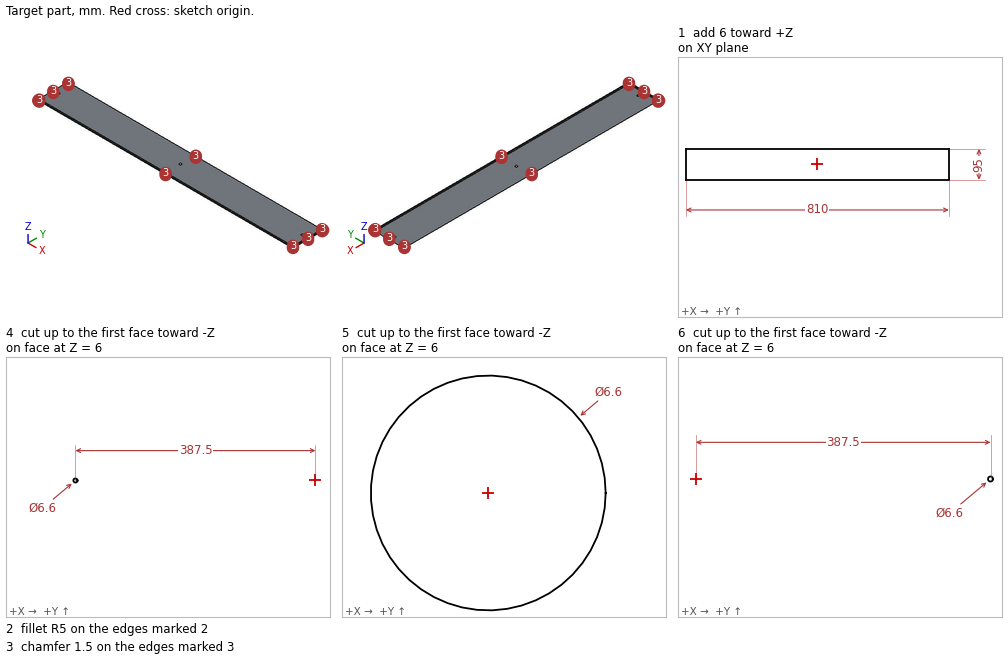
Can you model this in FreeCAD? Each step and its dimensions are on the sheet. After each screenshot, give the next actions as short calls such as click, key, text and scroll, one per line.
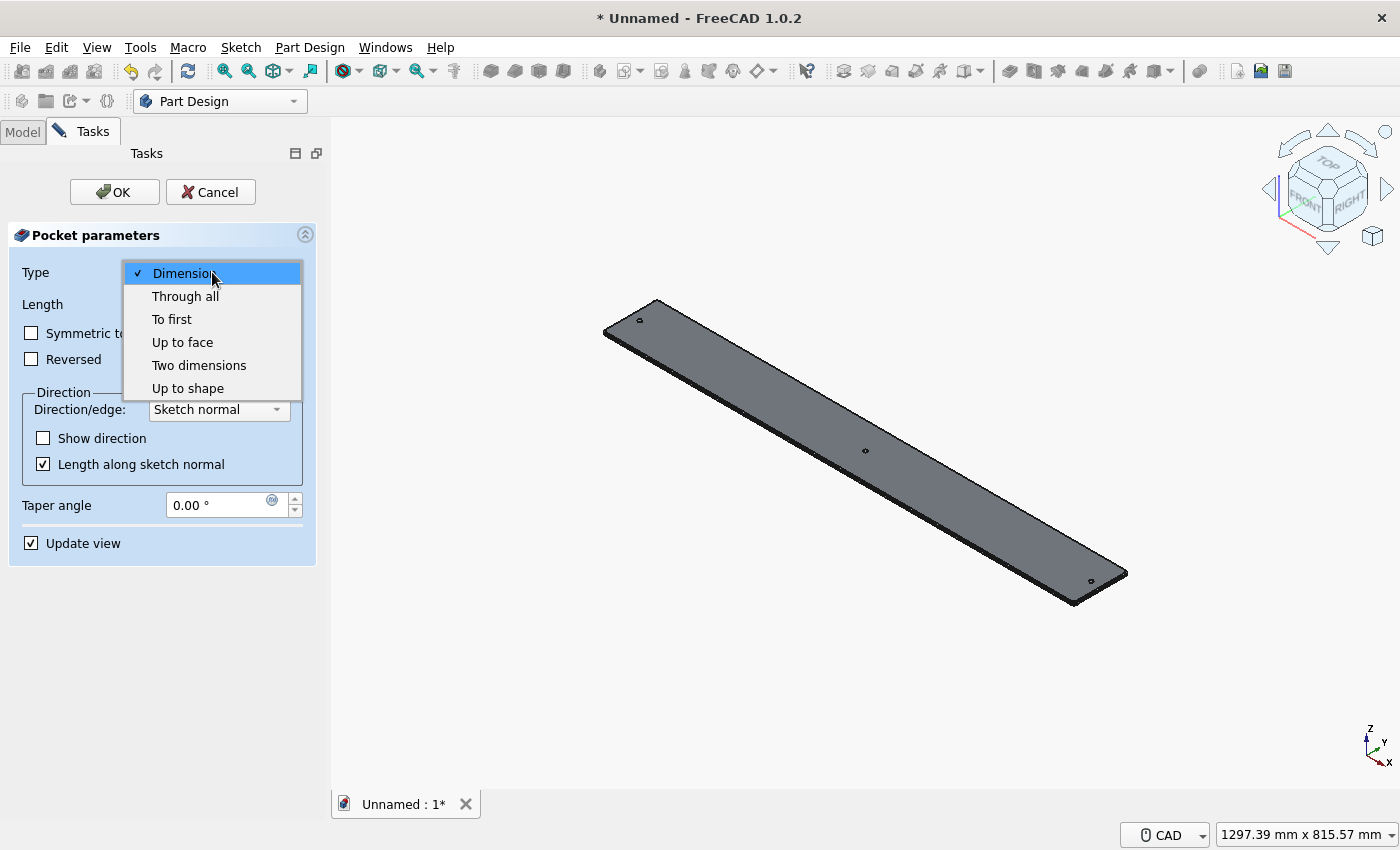
click(212, 320)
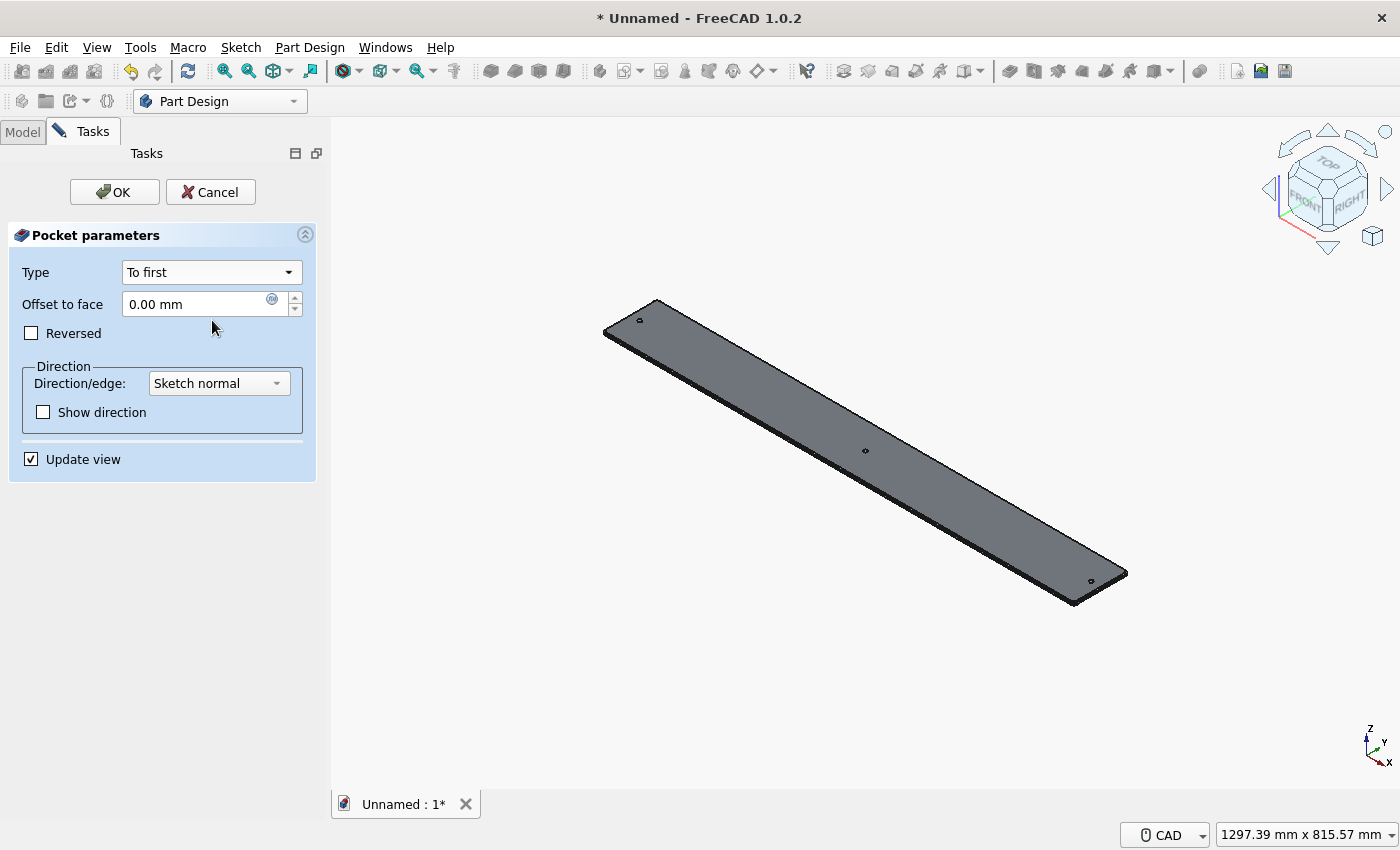
click(115, 192)